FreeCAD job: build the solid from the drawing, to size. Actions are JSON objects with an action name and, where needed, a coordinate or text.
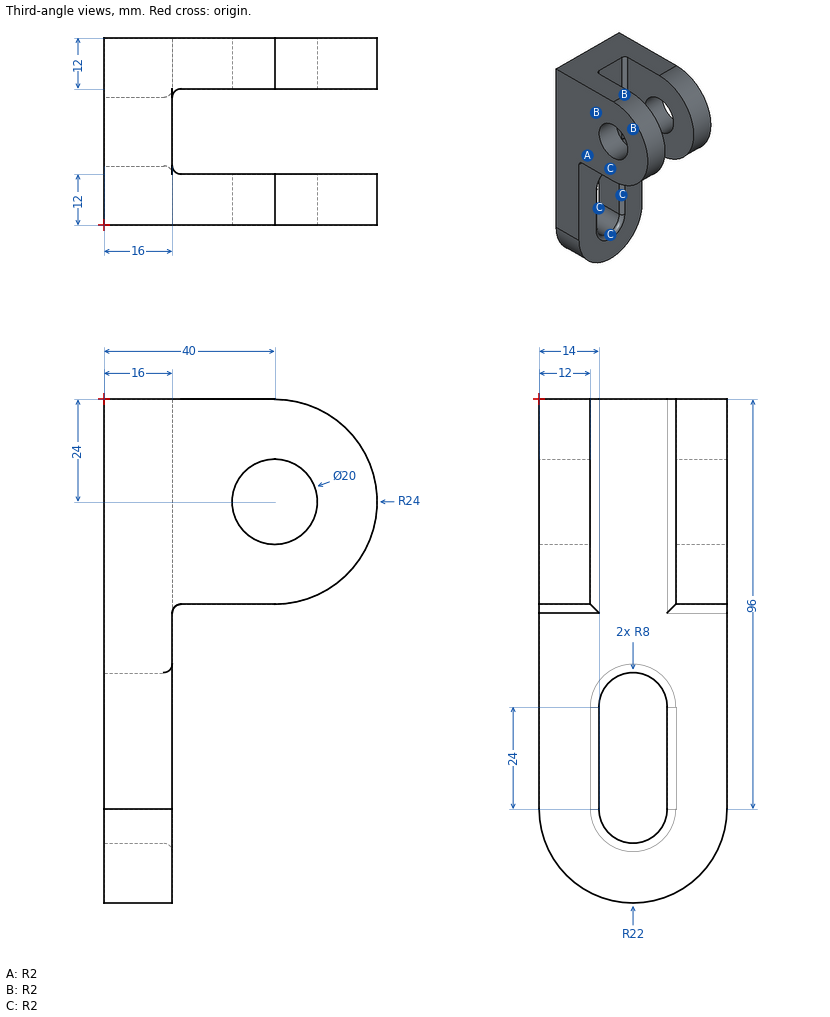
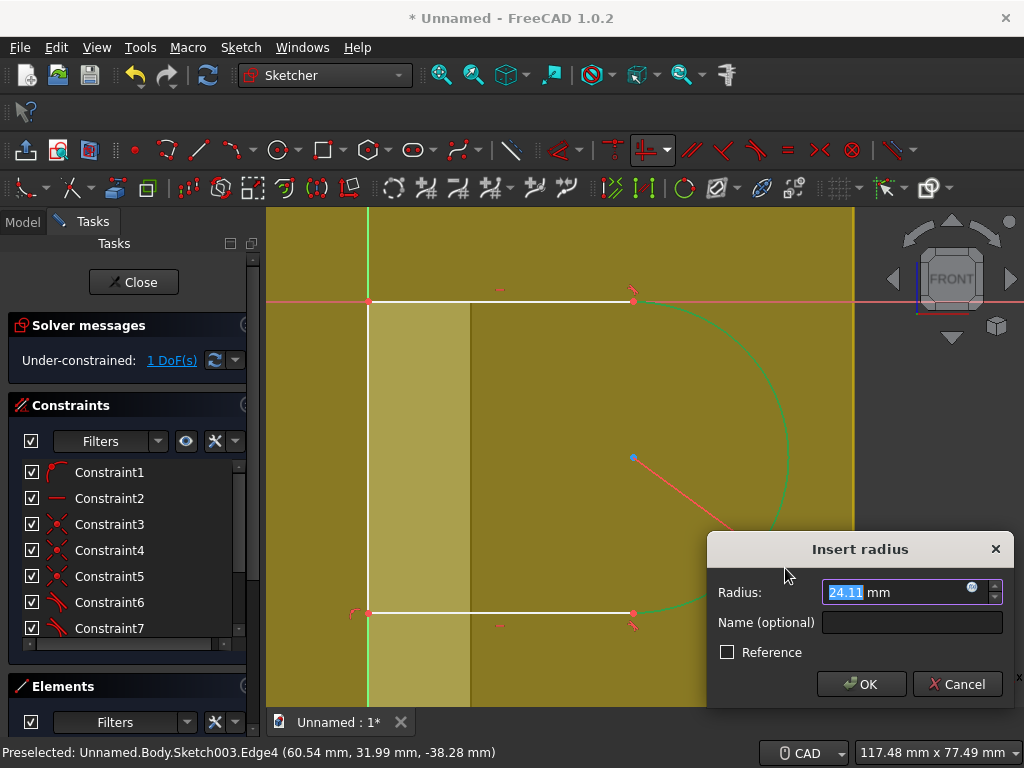
{"action": "type", "text": "24"}
{"action": "key", "text": "Return"}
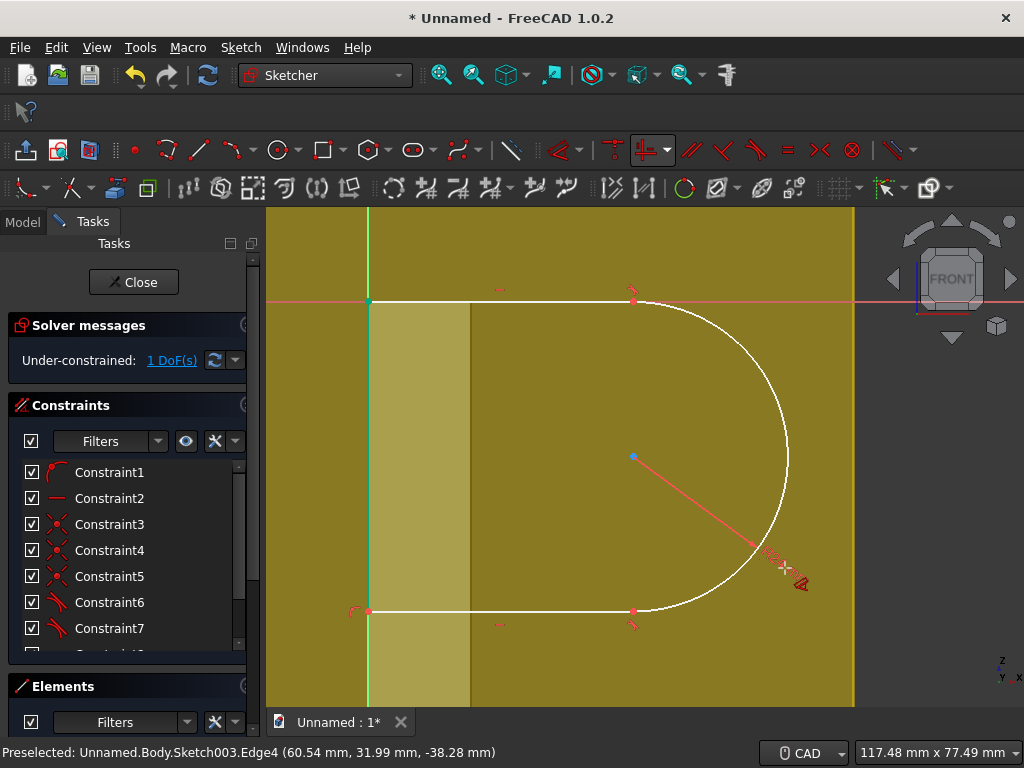
{"action": "left_click", "coordinate": [554, 612]}
{"action": "left_click", "coordinate": [501, 646]}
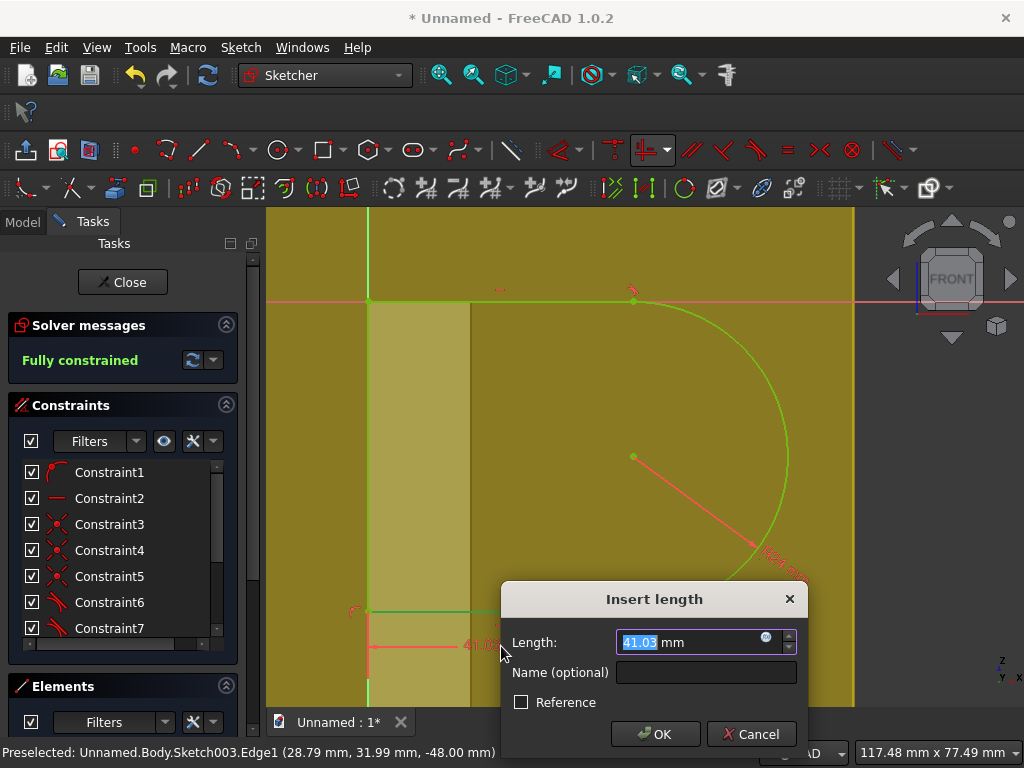
{"action": "type", "text": "40"}
{"action": "key", "text": "Return"}
{"action": "key", "text": "Escape"}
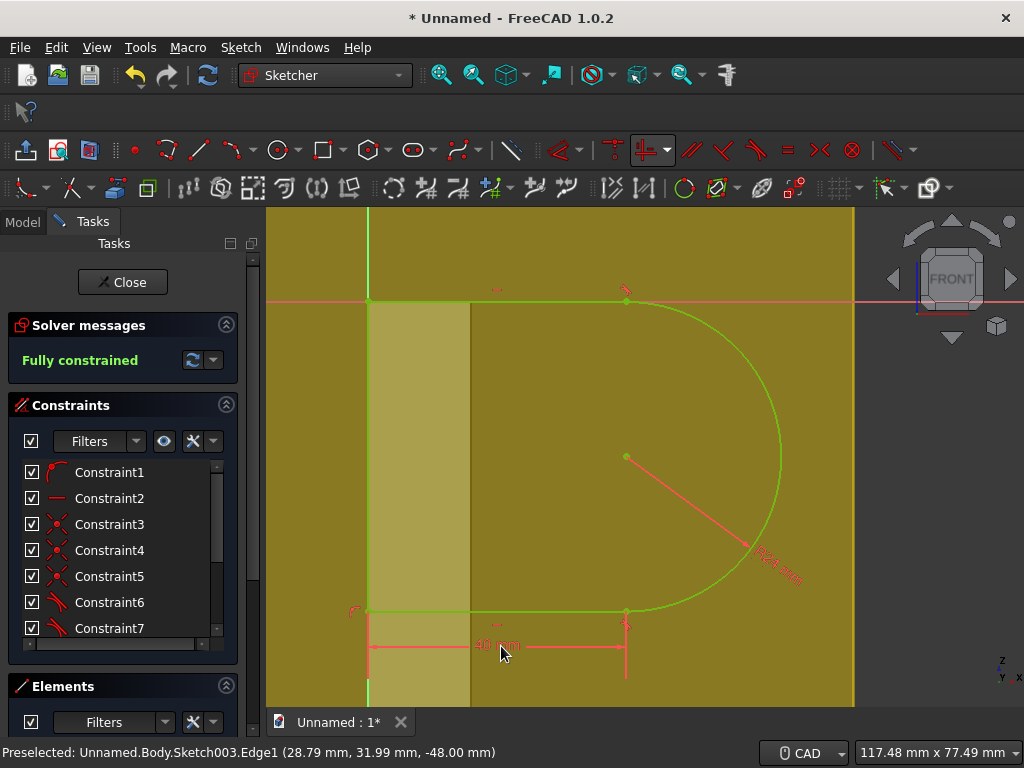
{"action": "left_click", "coordinate": [123, 282]}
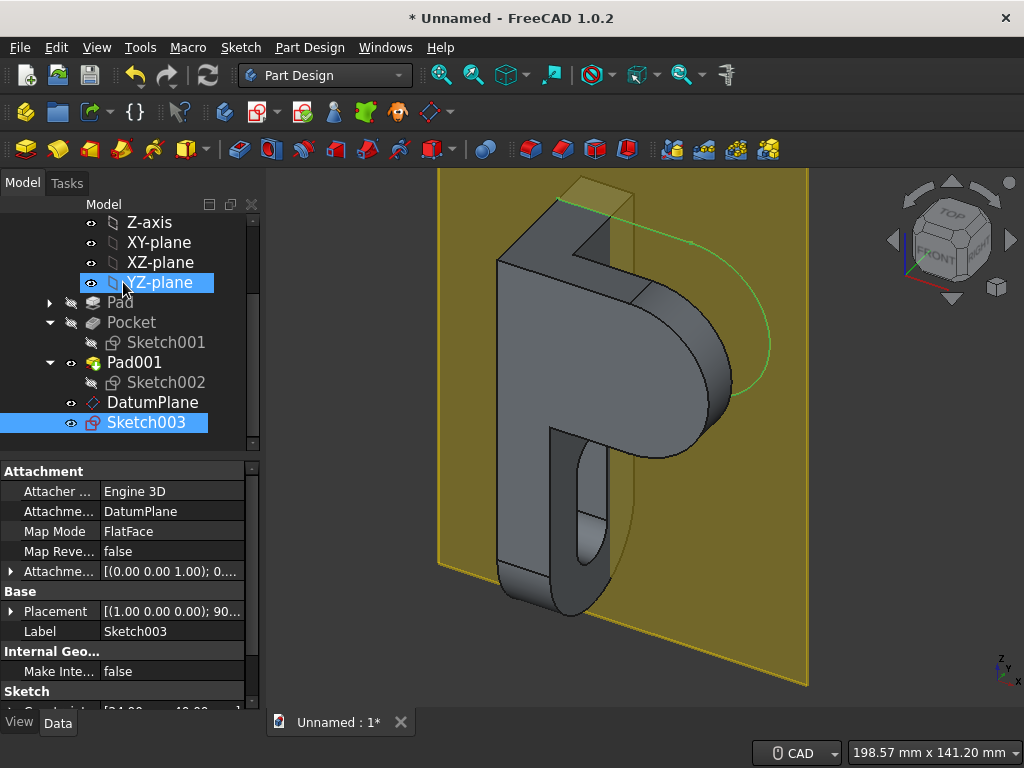
{"action": "left_click", "coordinate": [26, 150]}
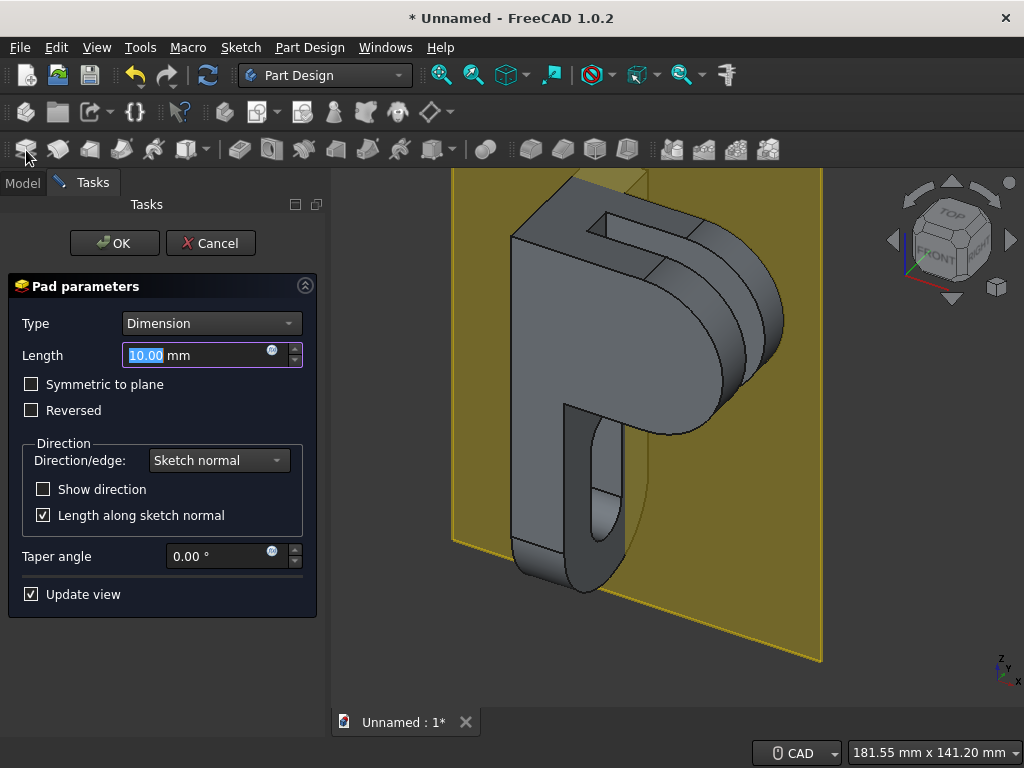
{"action": "type", "text": "12"}
{"action": "key", "text": "Tab"}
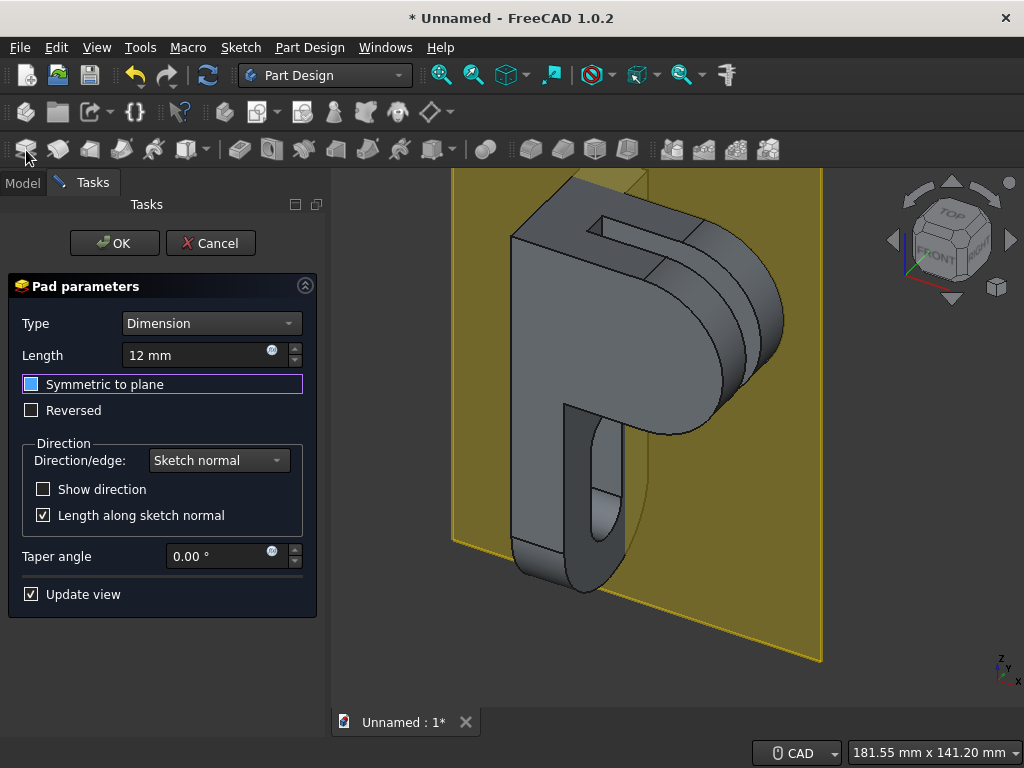
{"action": "left_click", "coordinate": [30, 410]}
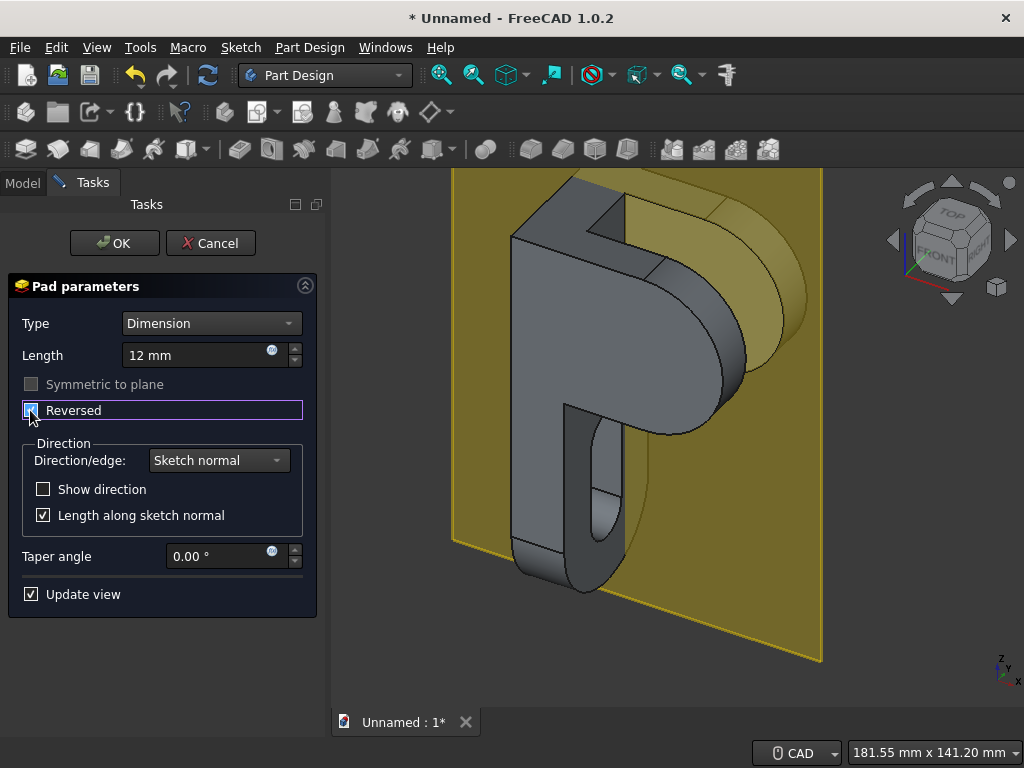
{"action": "left_click", "coordinate": [115, 243]}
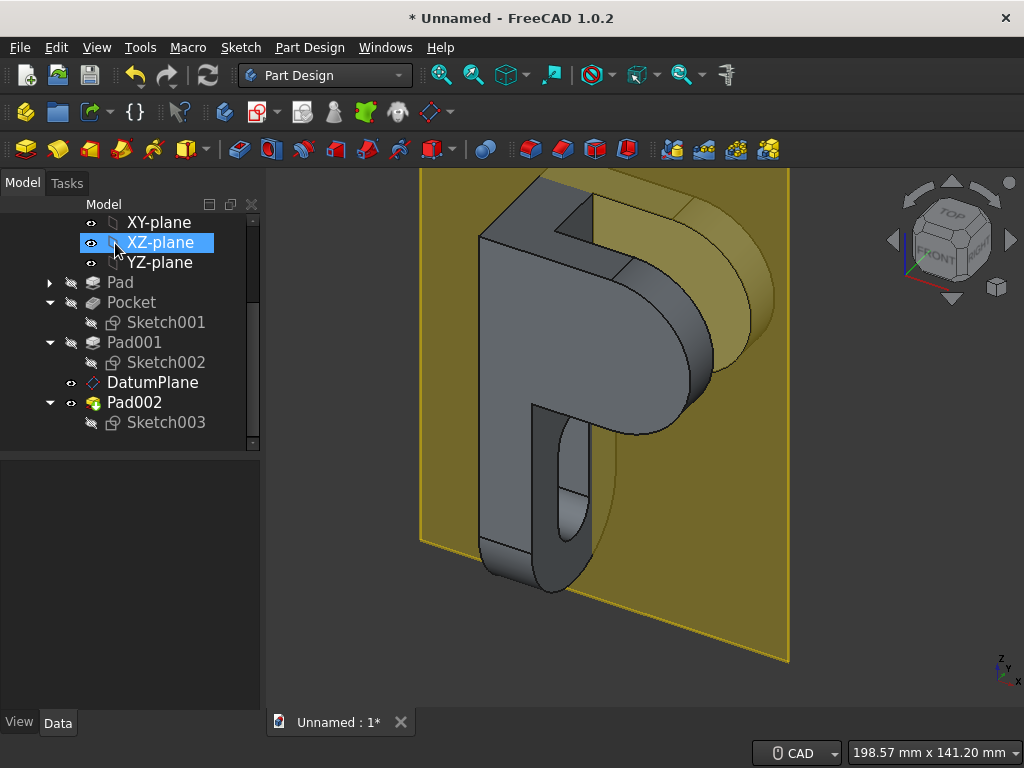
{"action": "left_click", "coordinate": [116, 383]}
{"action": "key", "text": "space"}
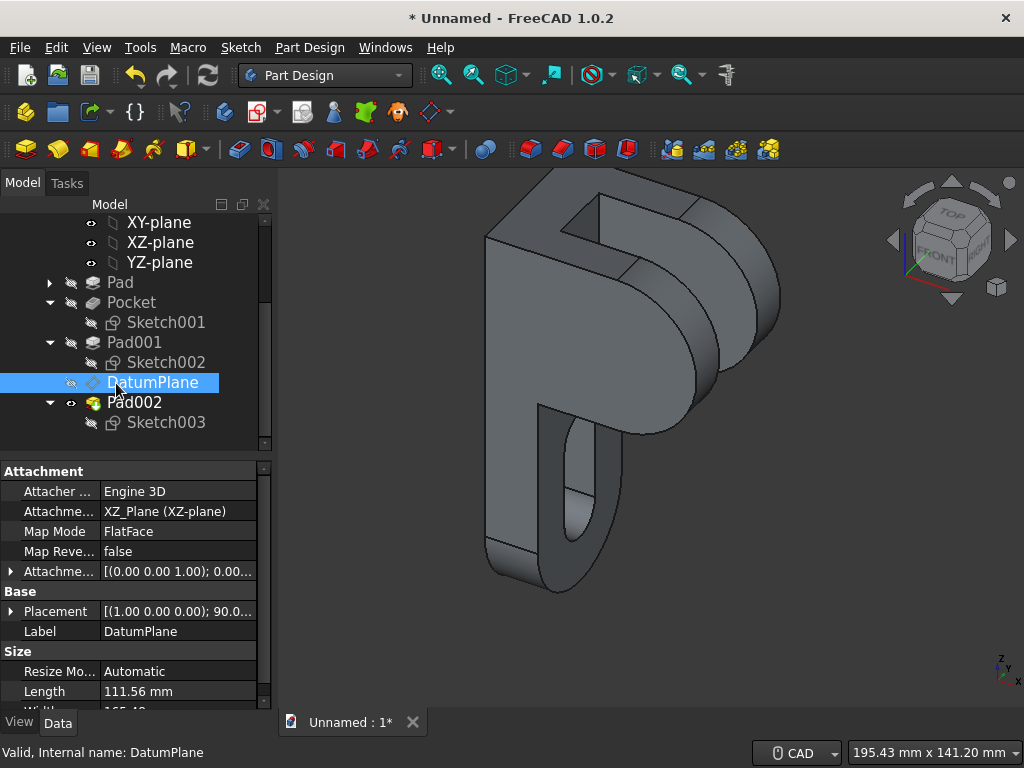
{"action": "key", "text": "v f"}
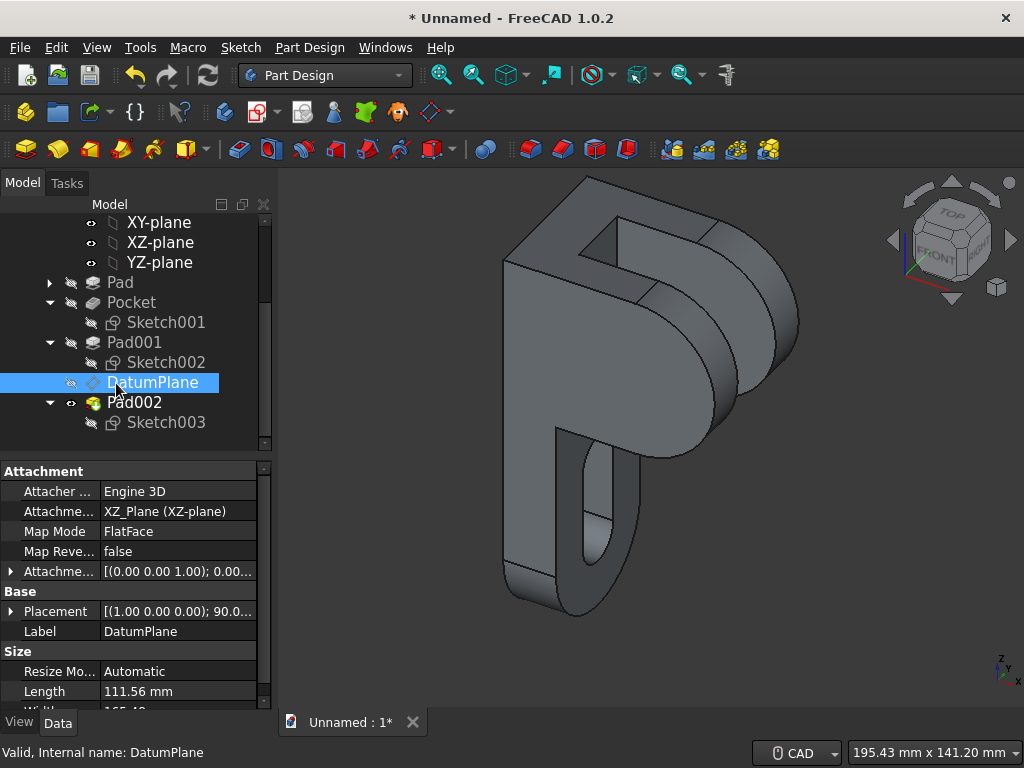
{"action": "key", "text": "4"}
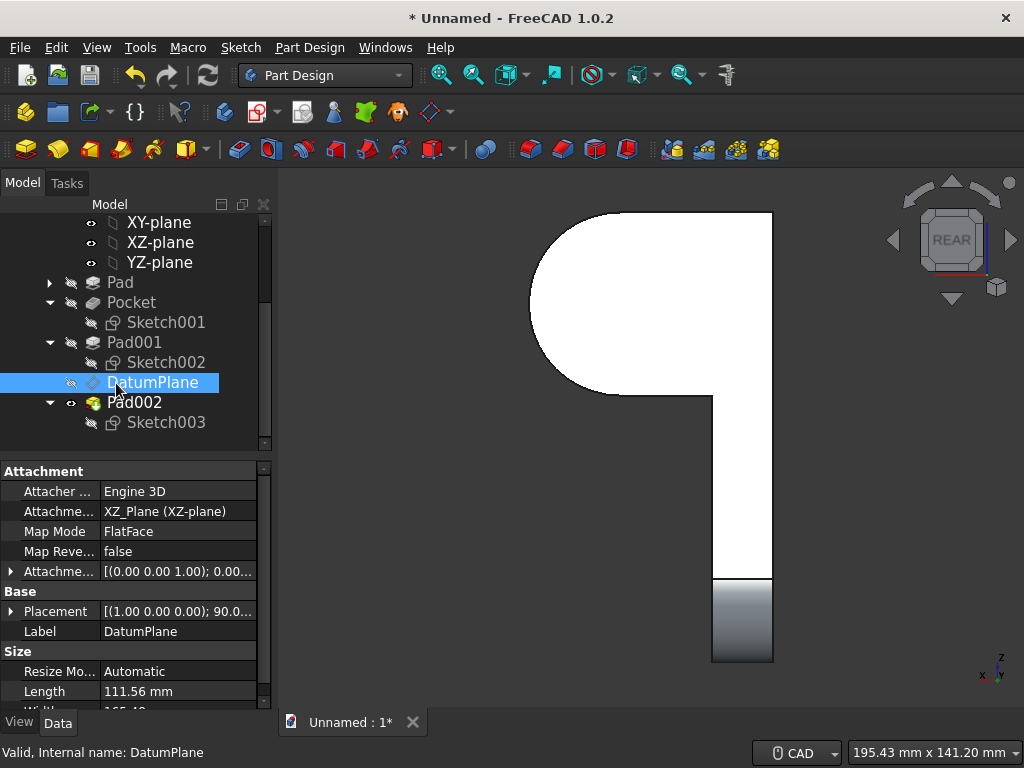
{"action": "left_click", "coordinate": [651, 290]}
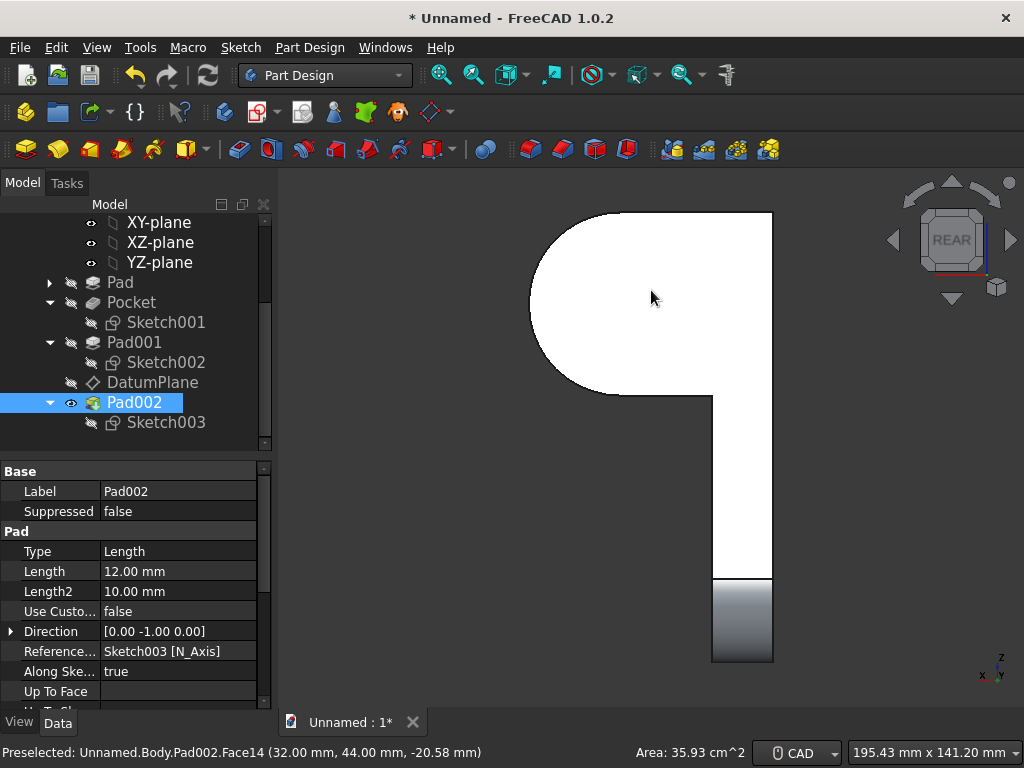
{"action": "left_click", "coordinate": [258, 112]}